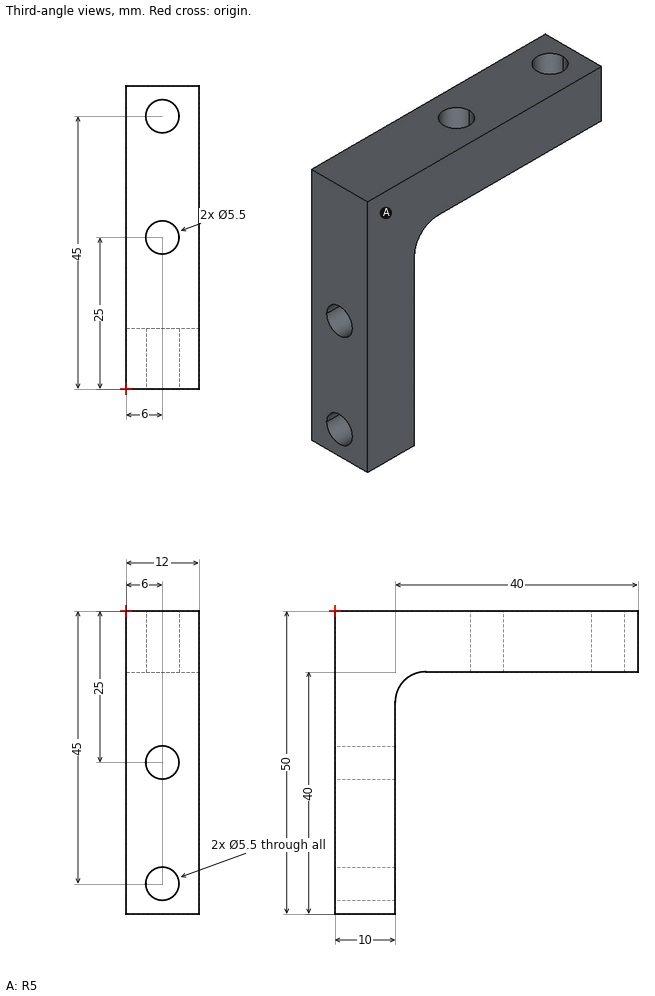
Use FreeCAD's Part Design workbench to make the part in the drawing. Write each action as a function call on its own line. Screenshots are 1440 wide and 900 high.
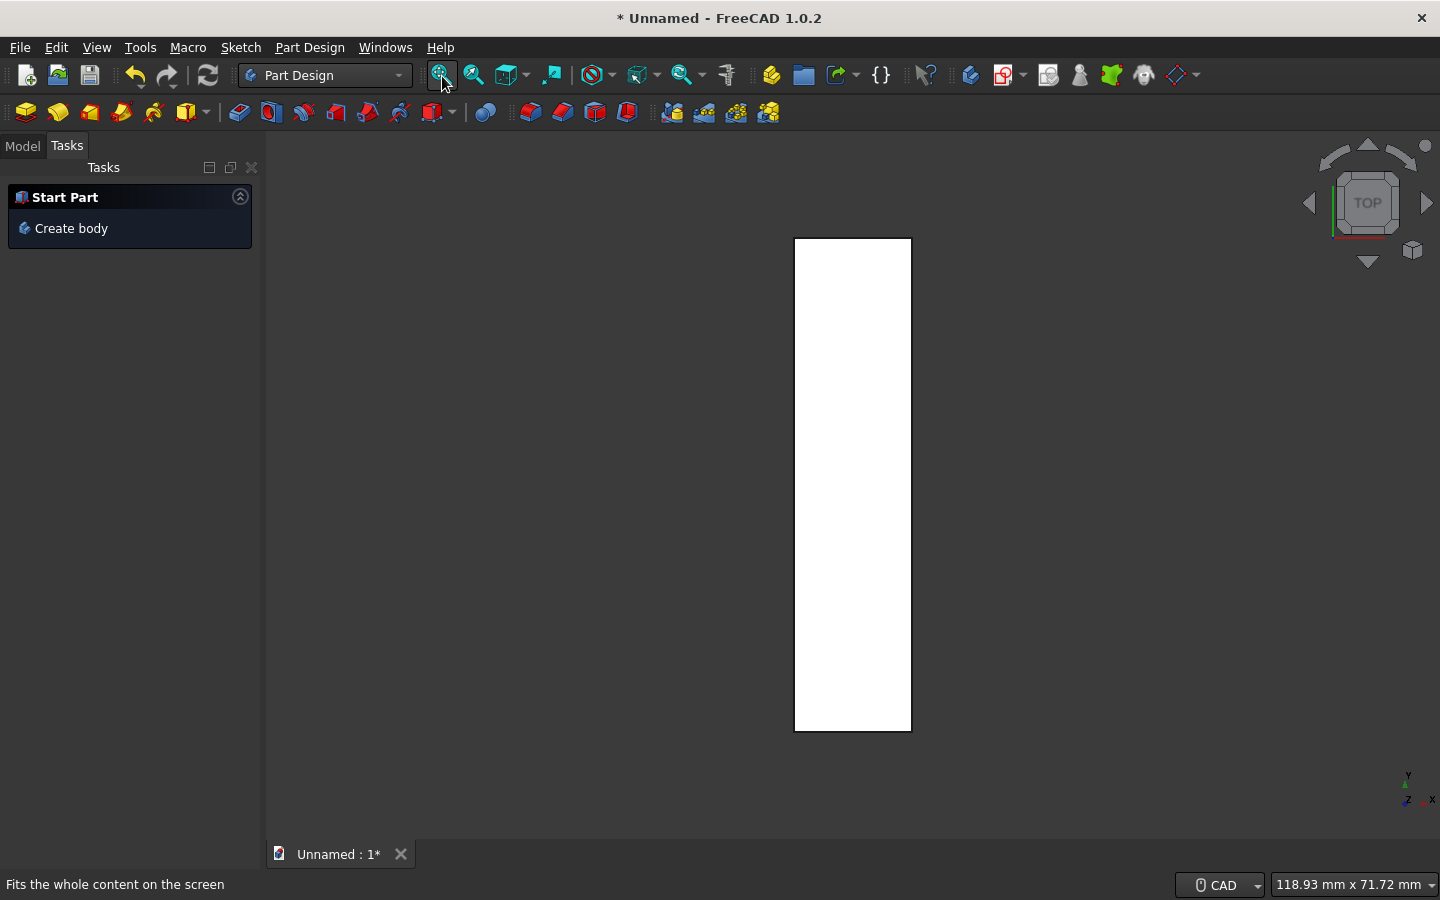
key(1)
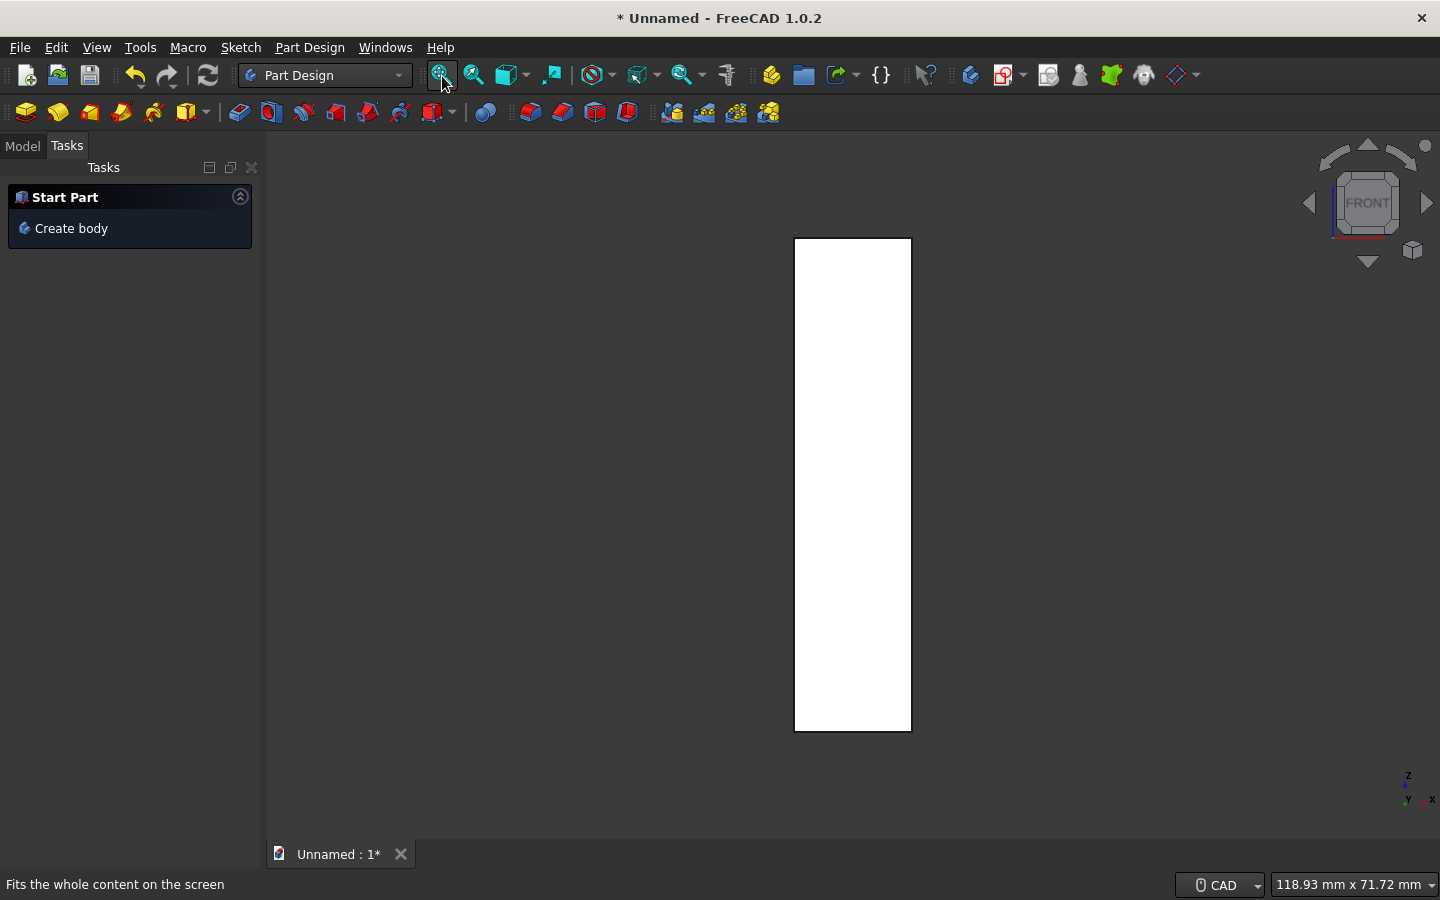
key(3)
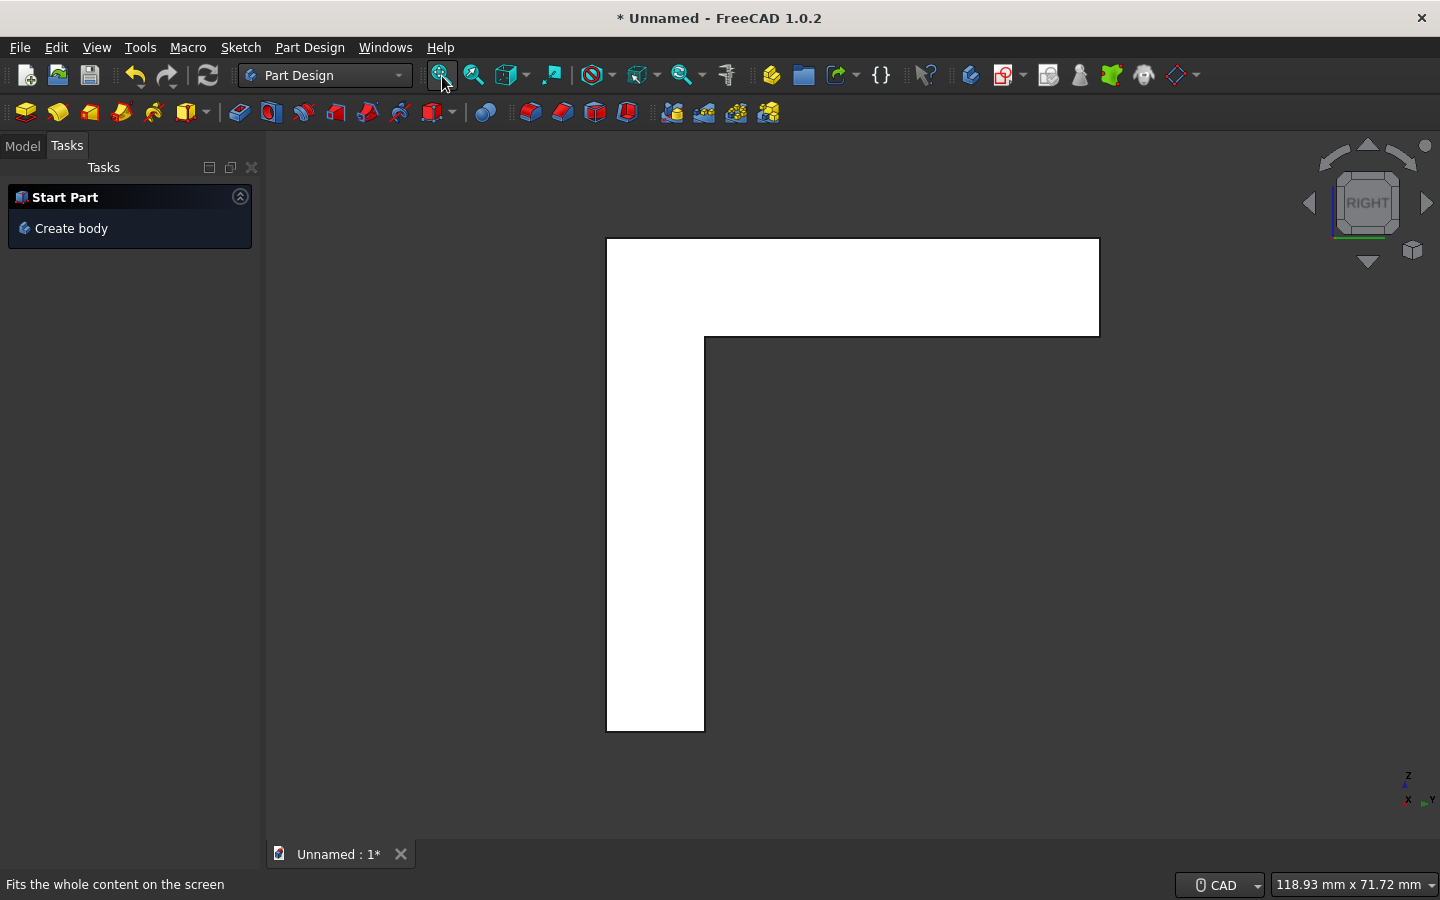
key(5)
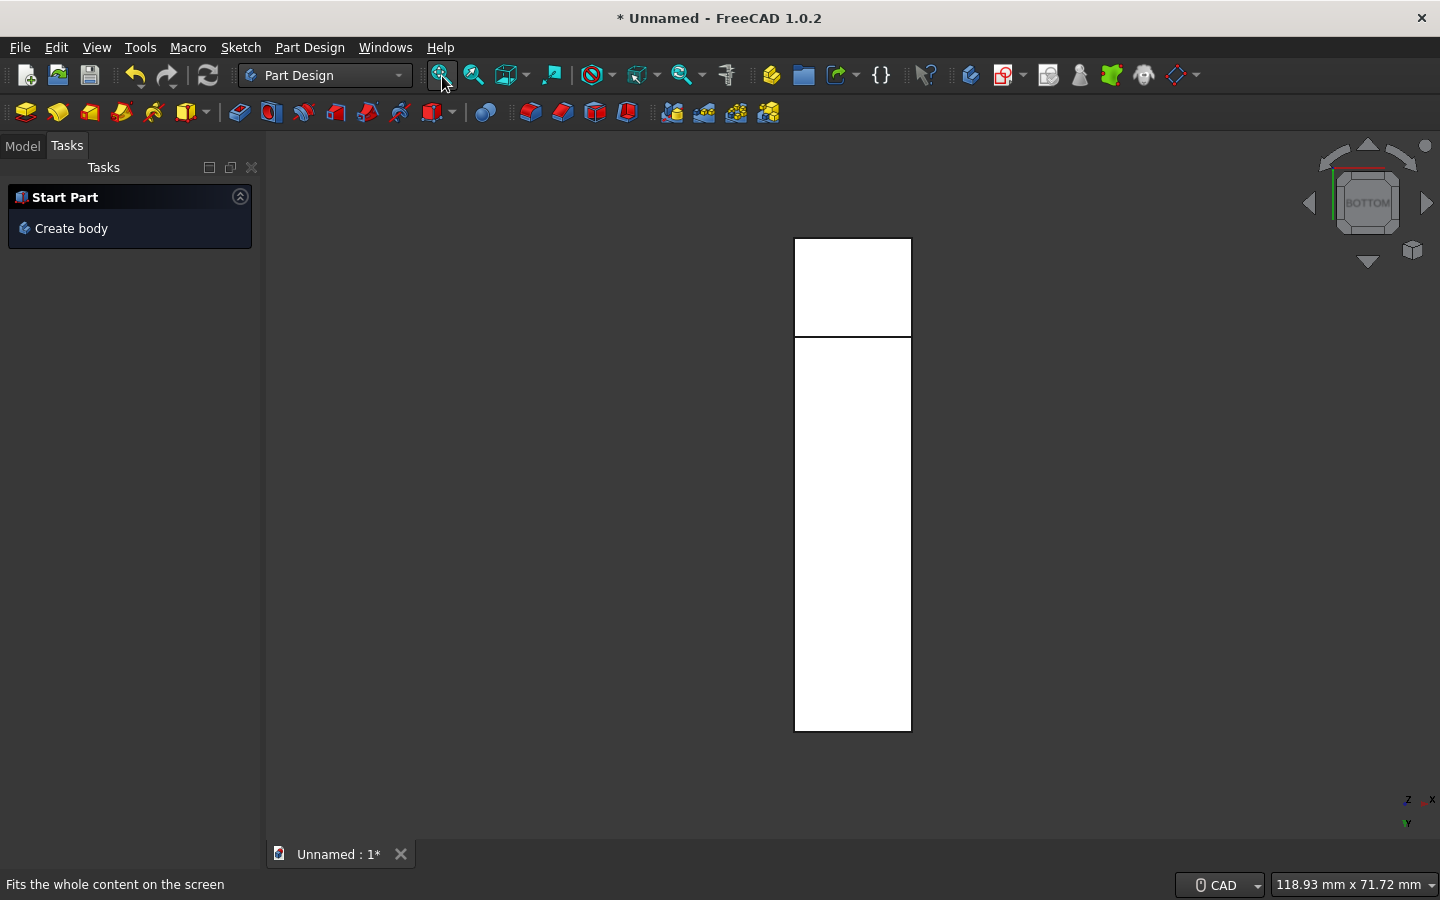
key(4)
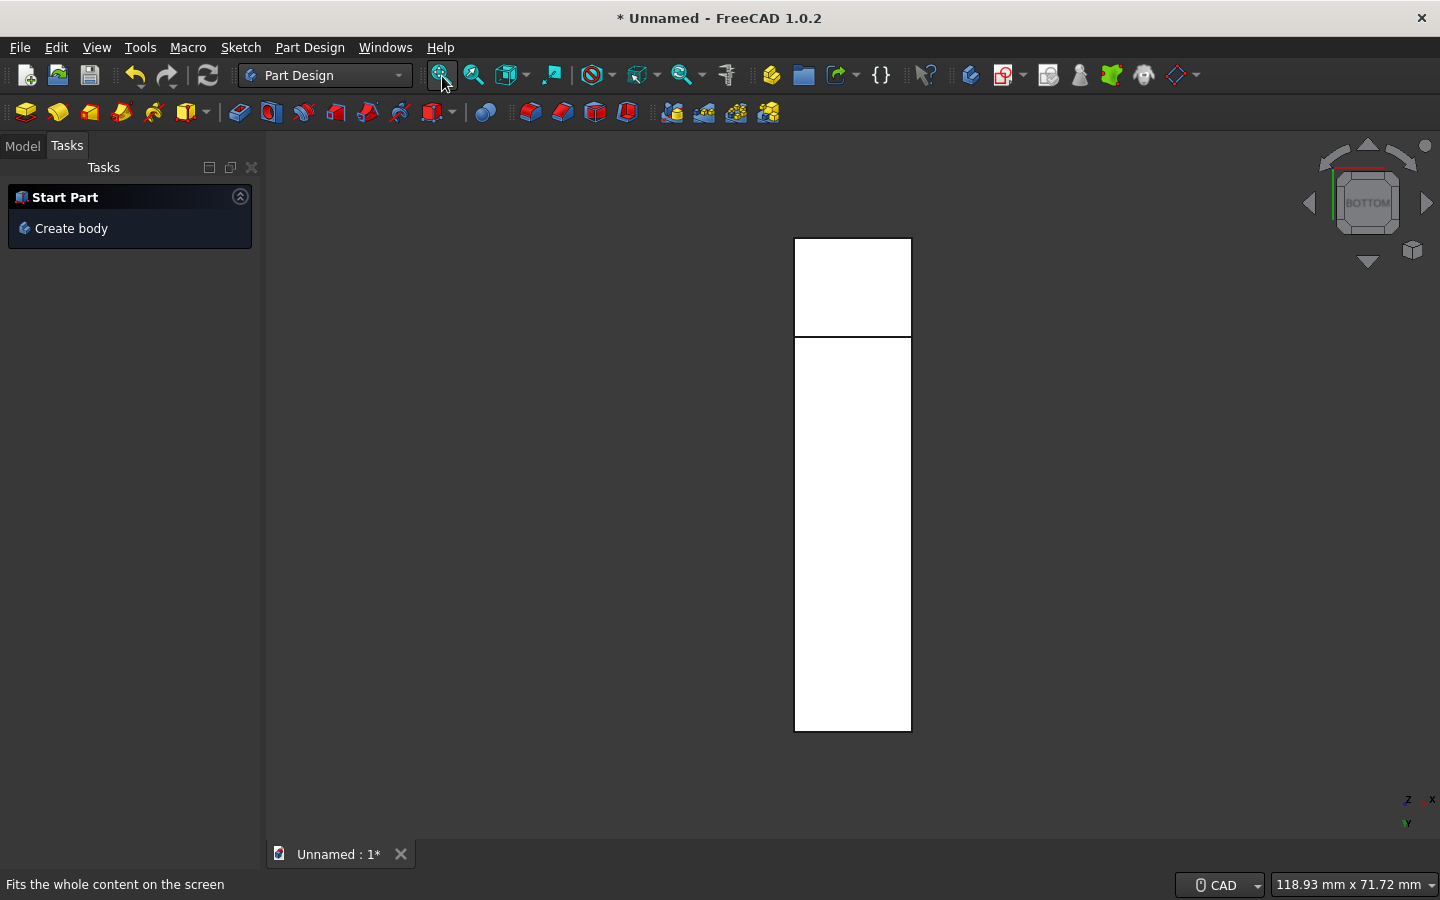
key(6)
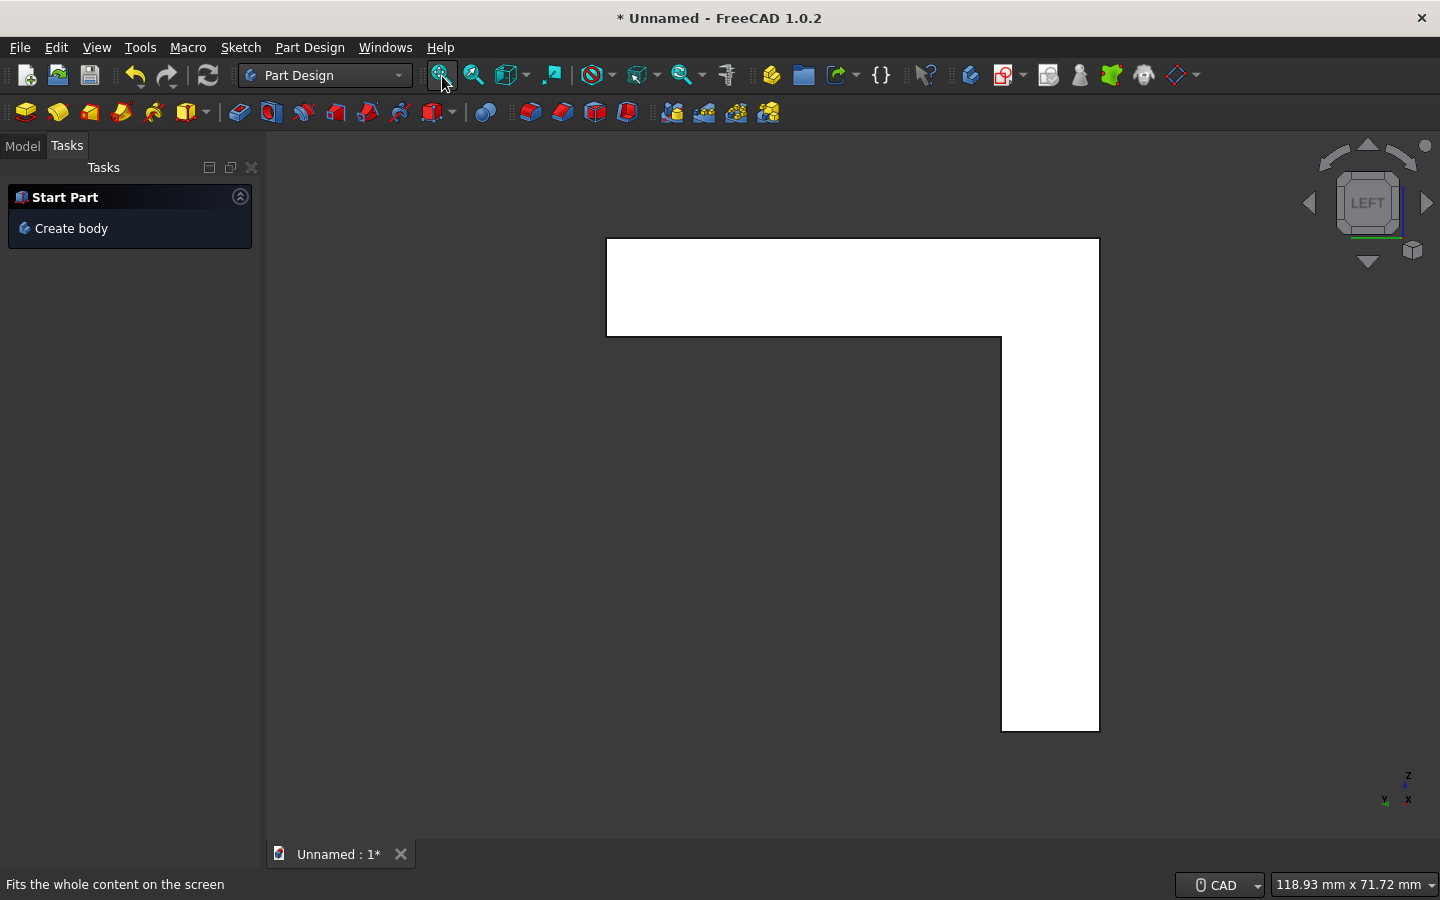
key(v)
key(3)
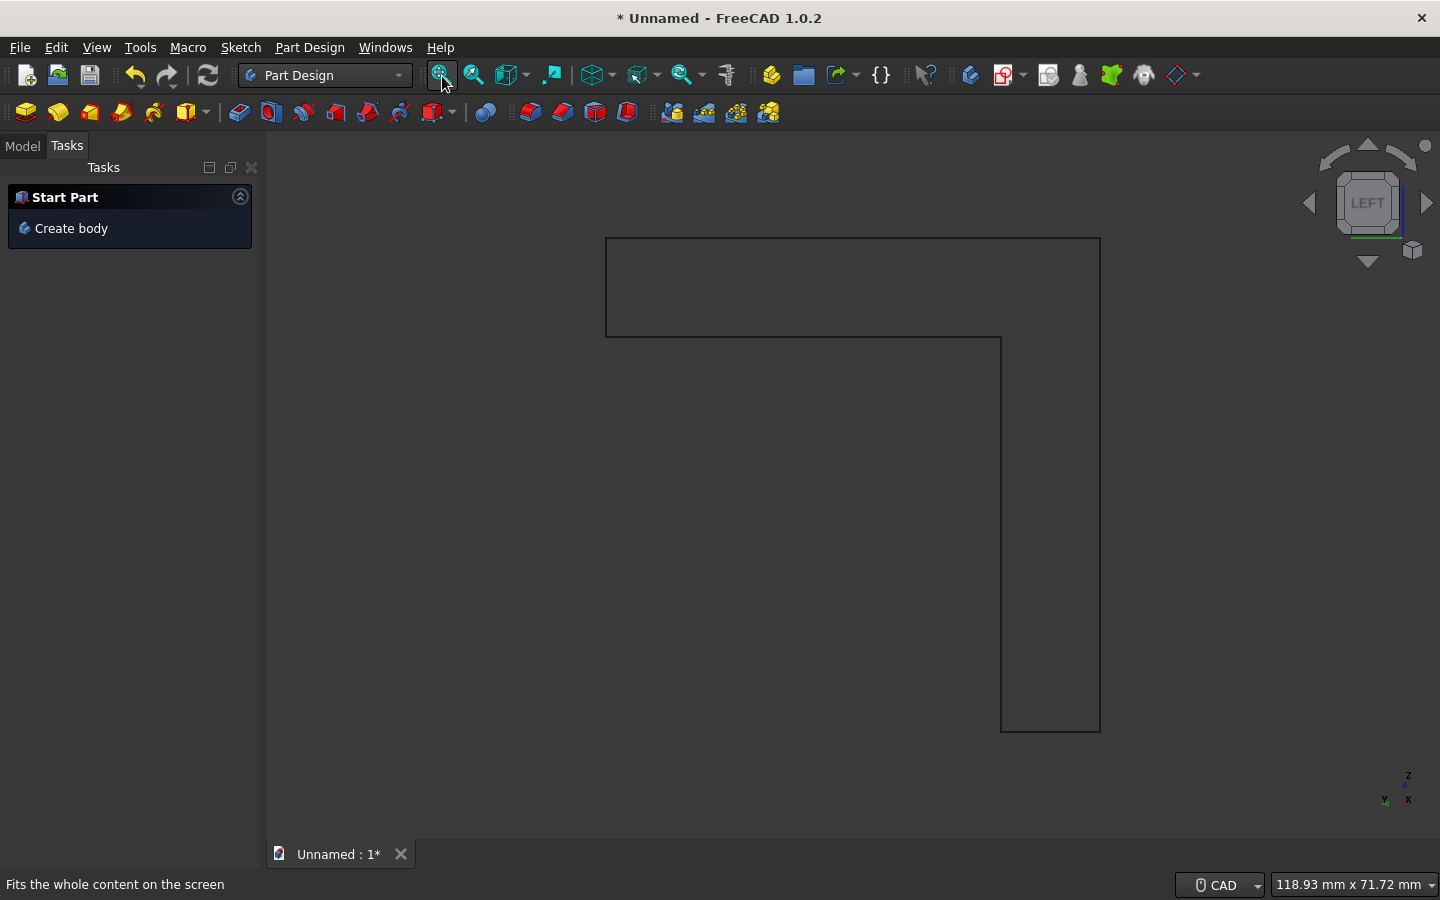
key(0)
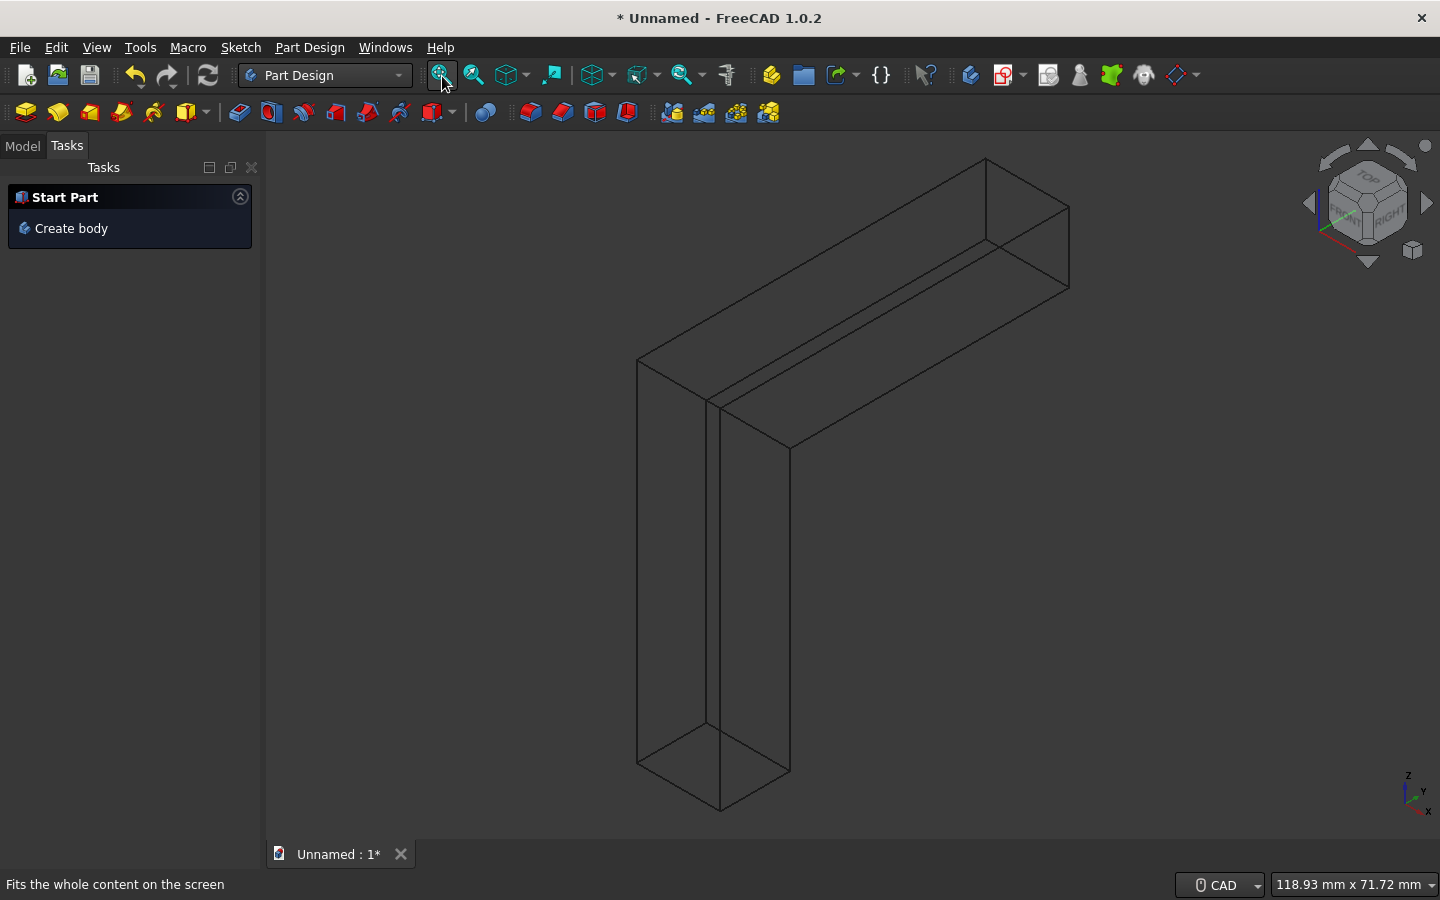
click(748, 424)